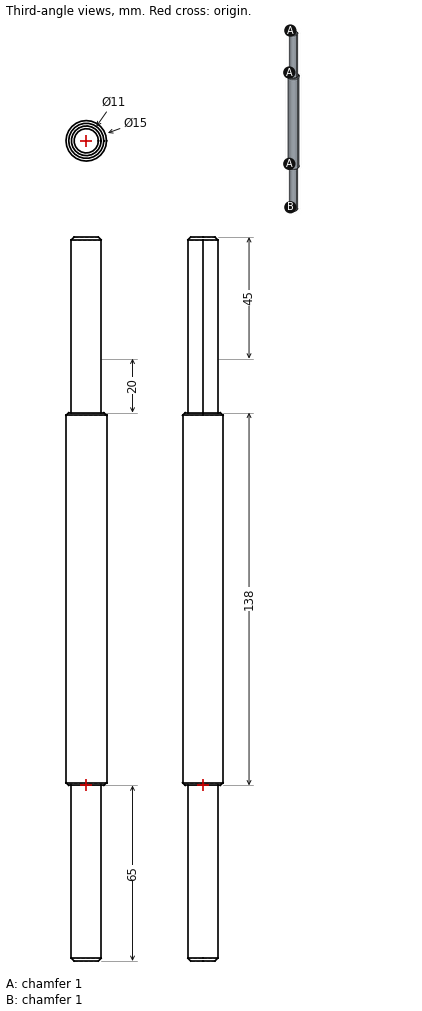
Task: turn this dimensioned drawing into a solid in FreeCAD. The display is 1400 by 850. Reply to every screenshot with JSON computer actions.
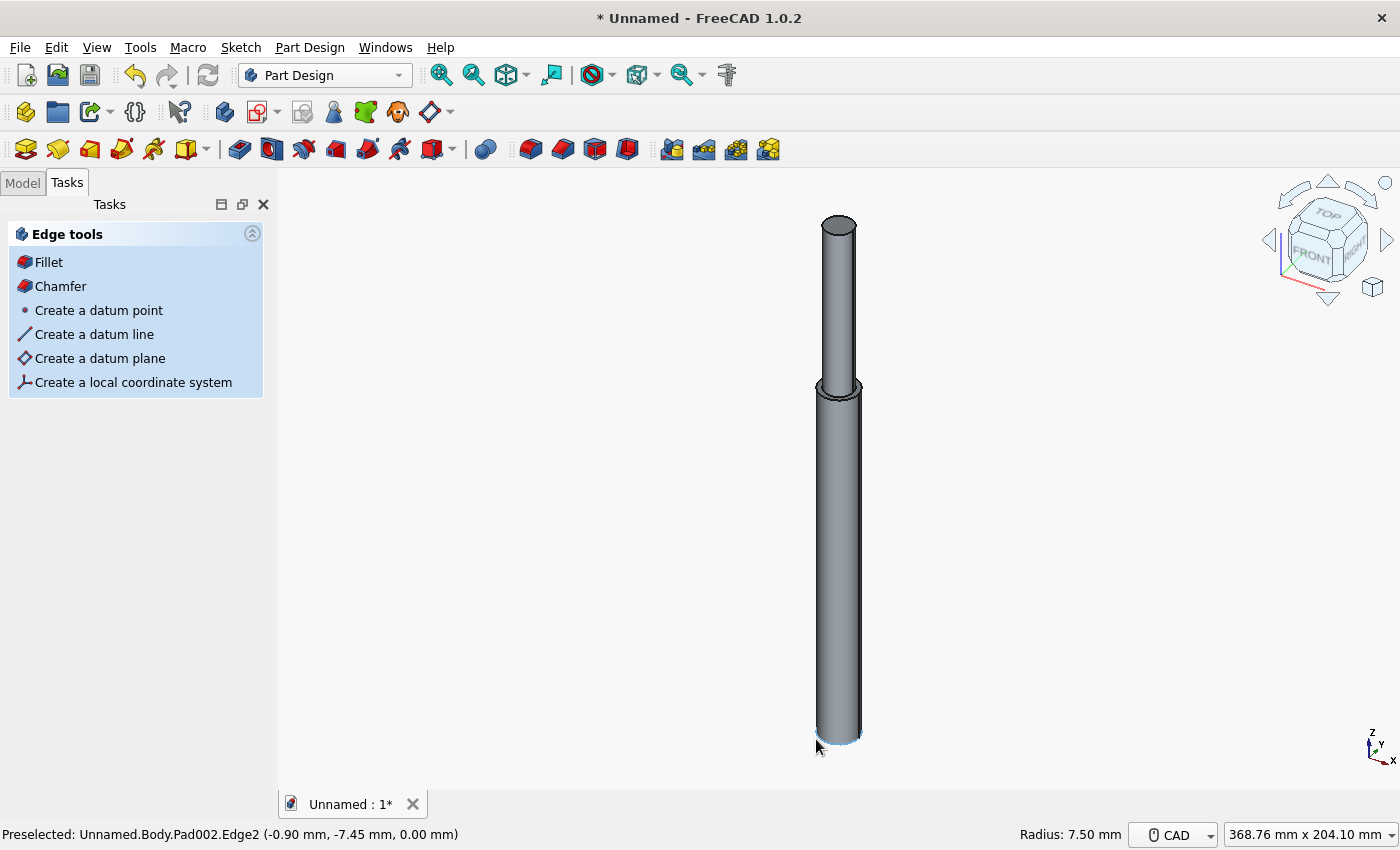
{"action": "left_click", "coordinate": [816, 388], "text": "ctrl"}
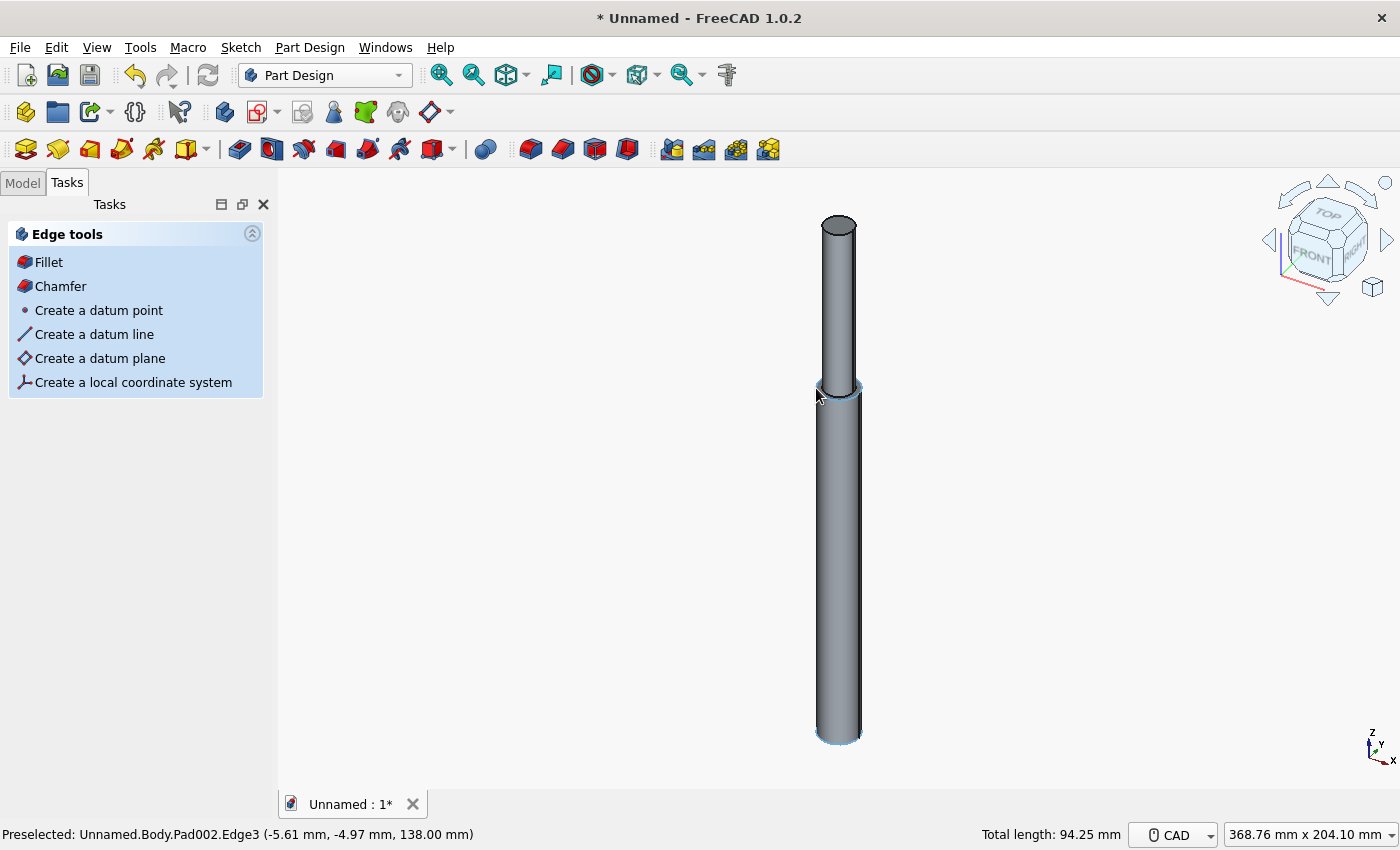
{"action": "left_click", "coordinate": [825, 220], "text": "ctrl"}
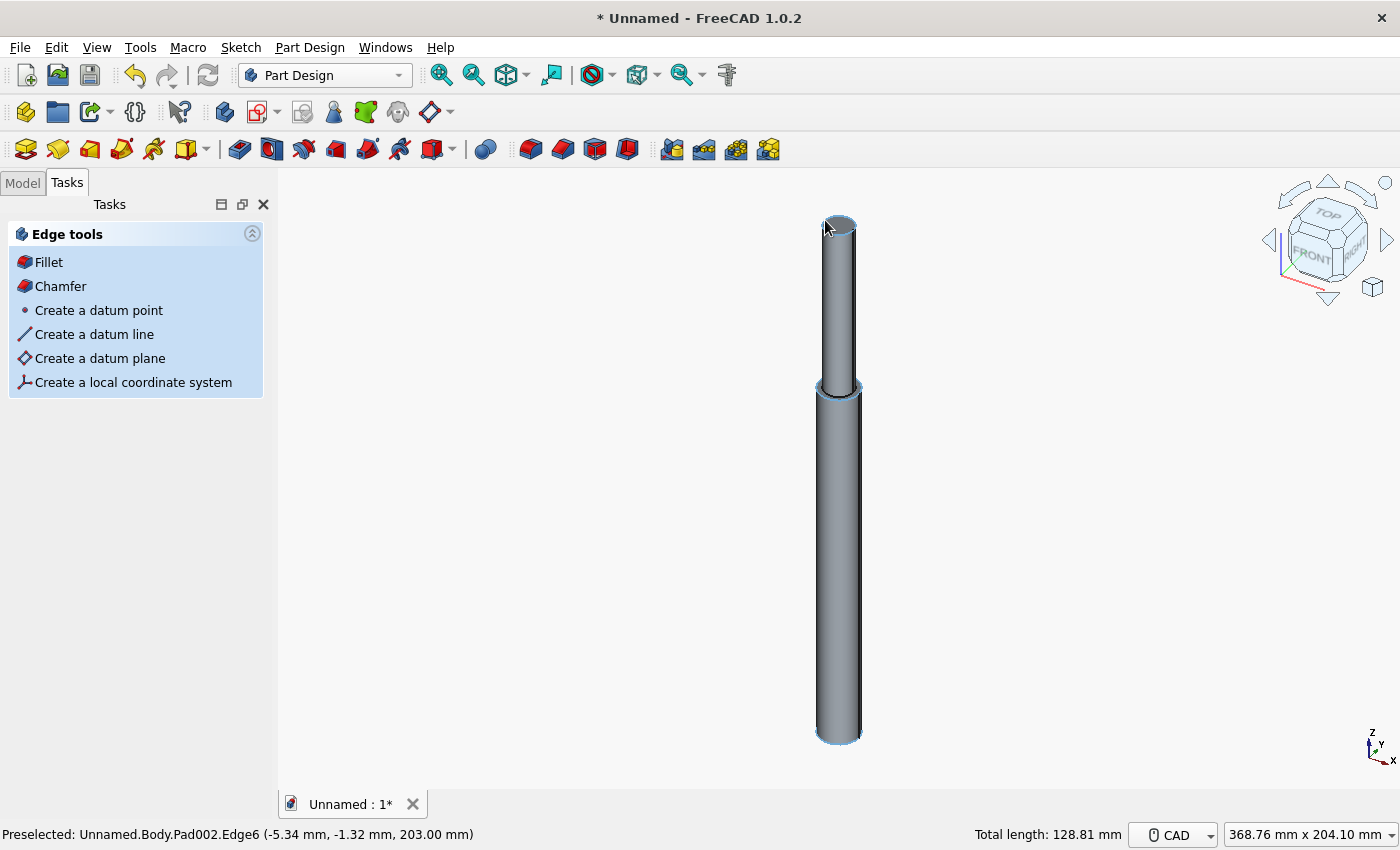
{"action": "left_click", "coordinate": [564, 150]}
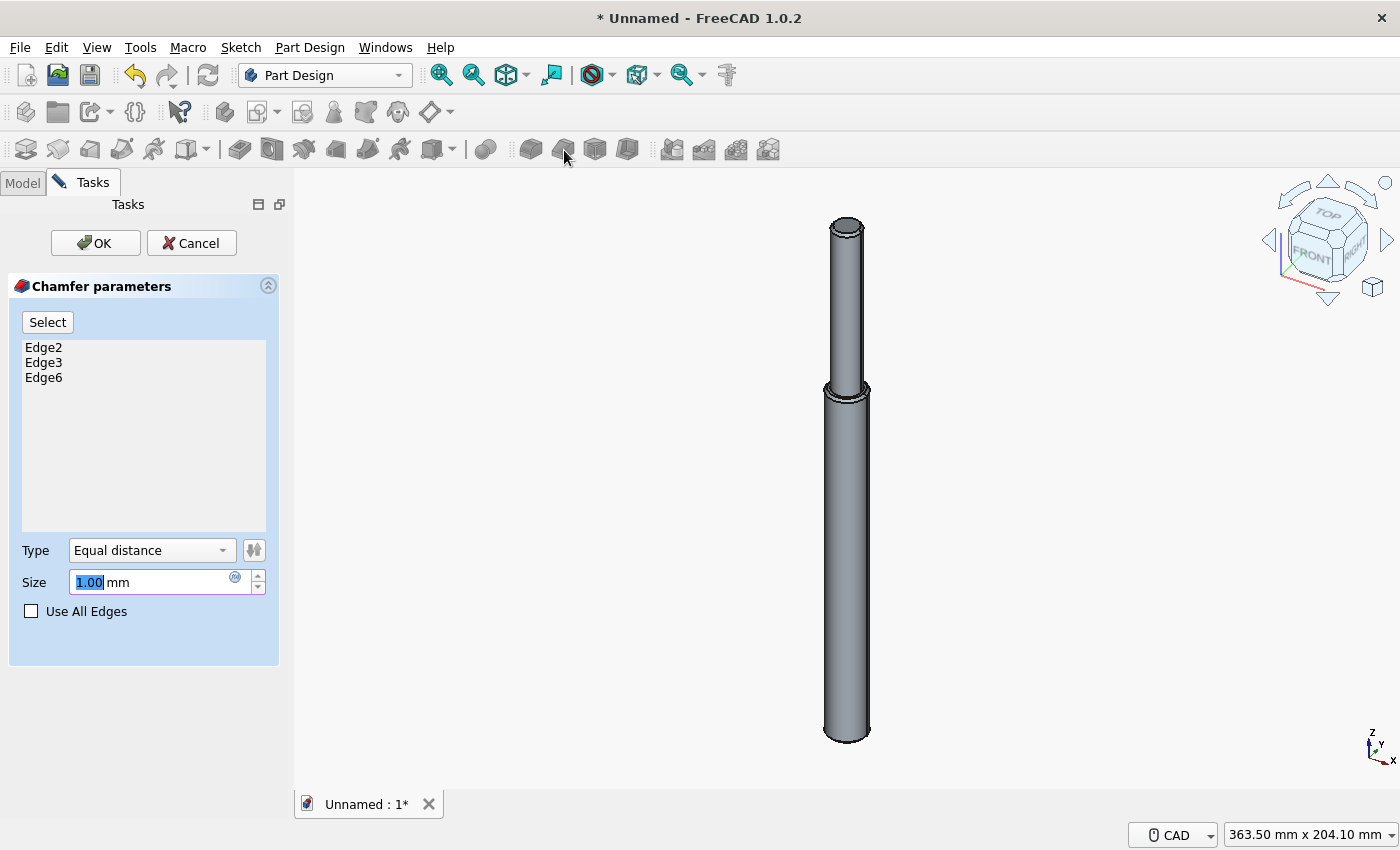
{"action": "type", "text": "1"}
{"action": "key", "text": "Tab"}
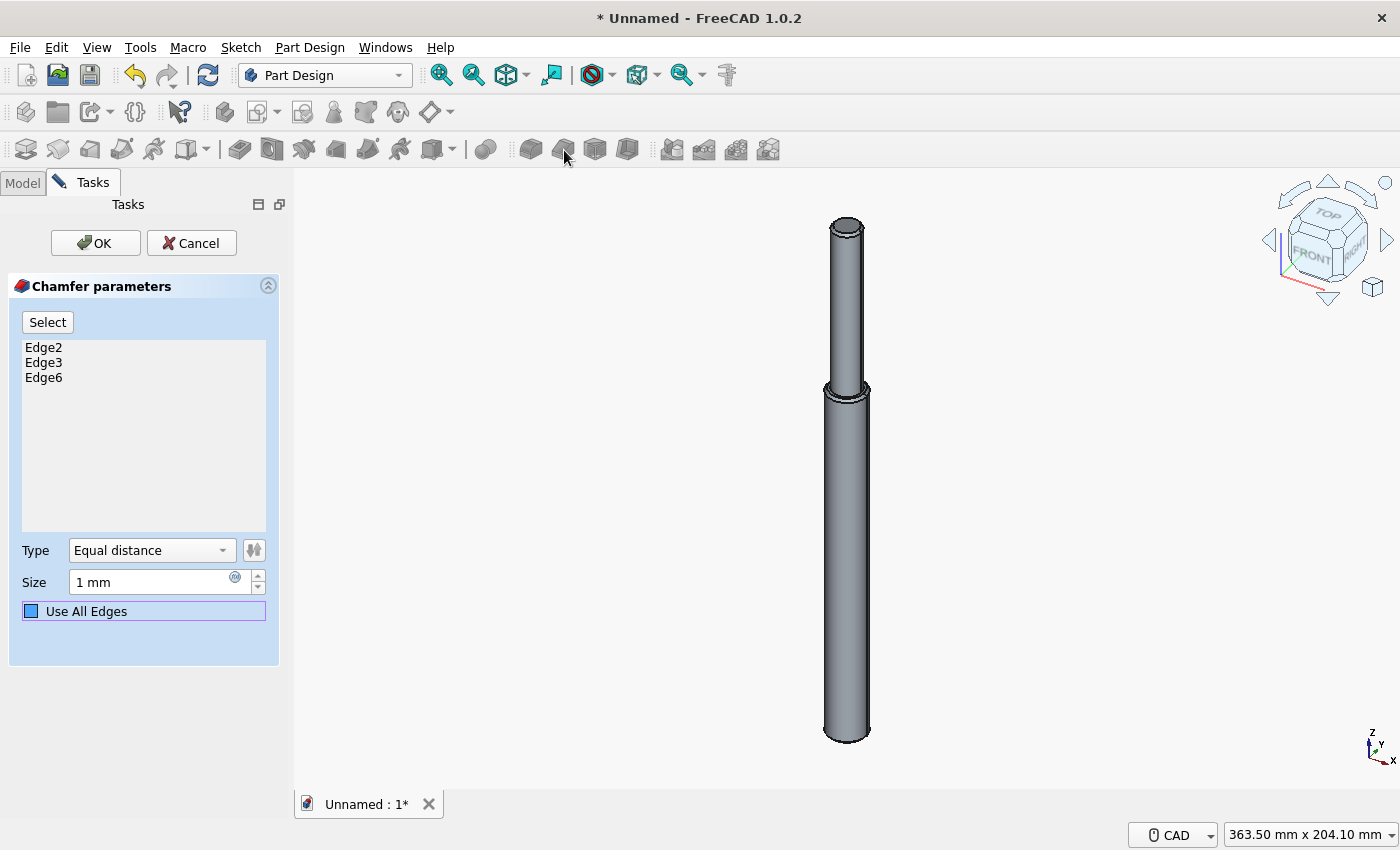
{"action": "left_click", "coordinate": [96, 243]}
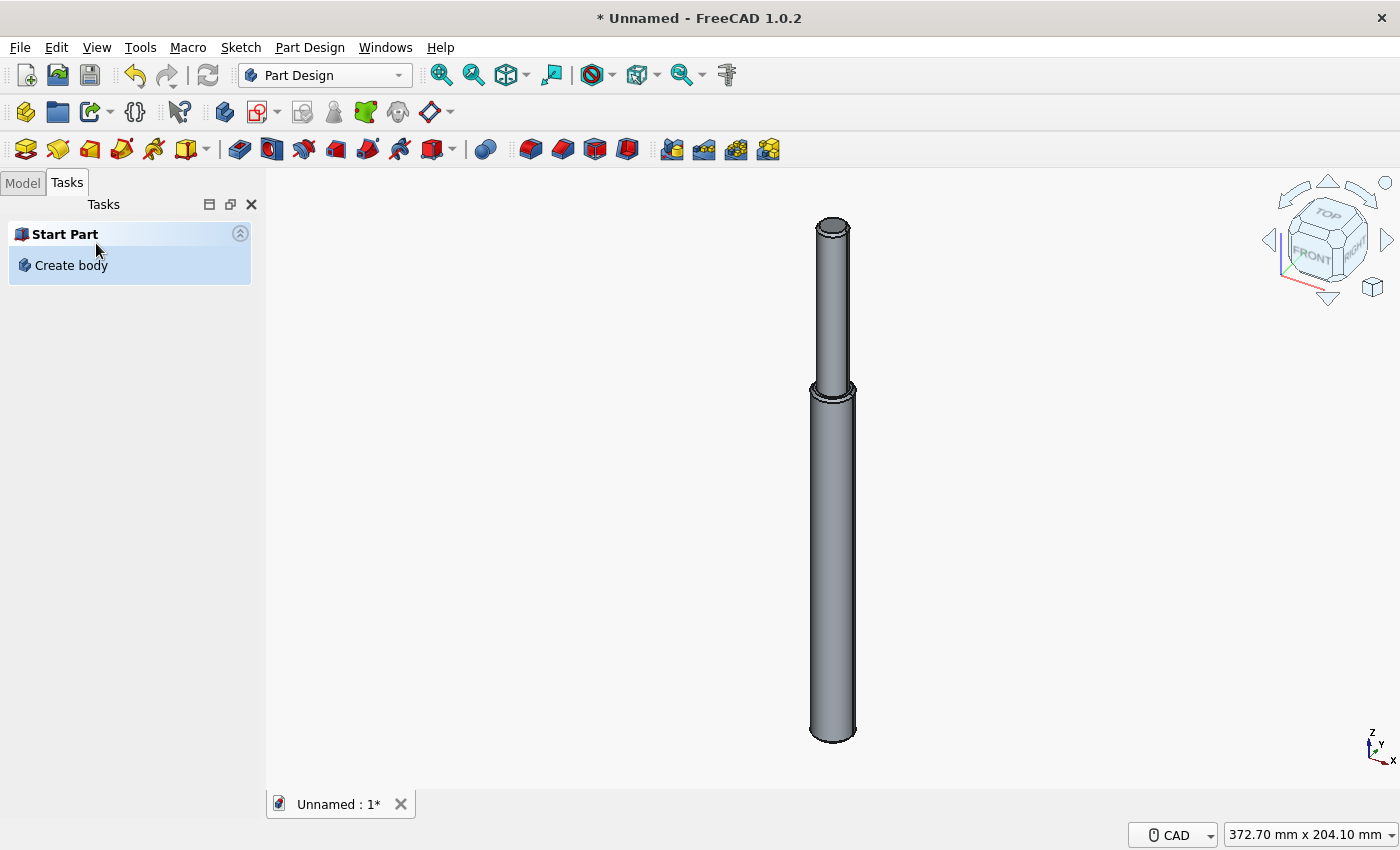
{"action": "left_click", "coordinate": [23, 182]}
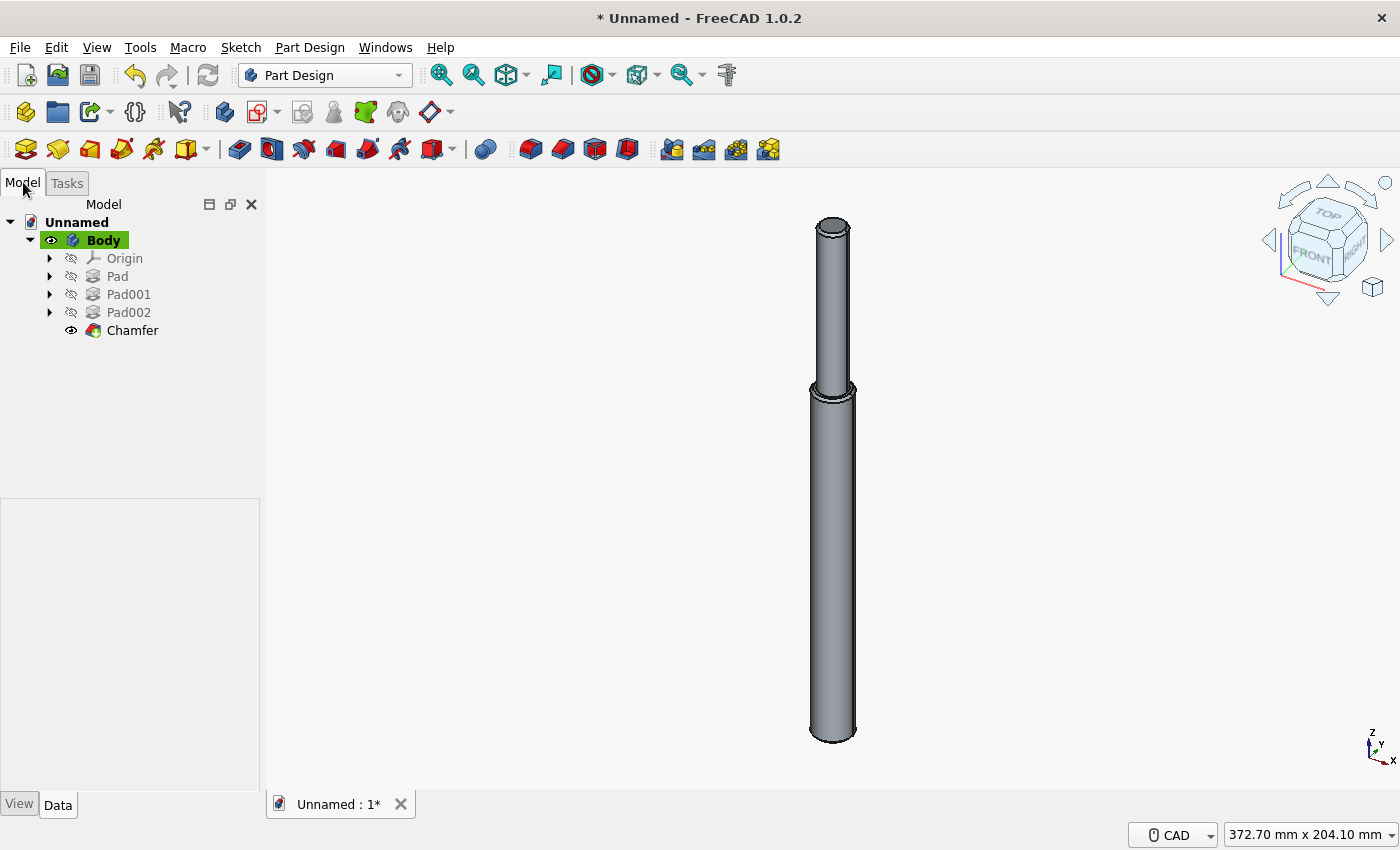
{"action": "left_click", "coordinate": [50, 258]}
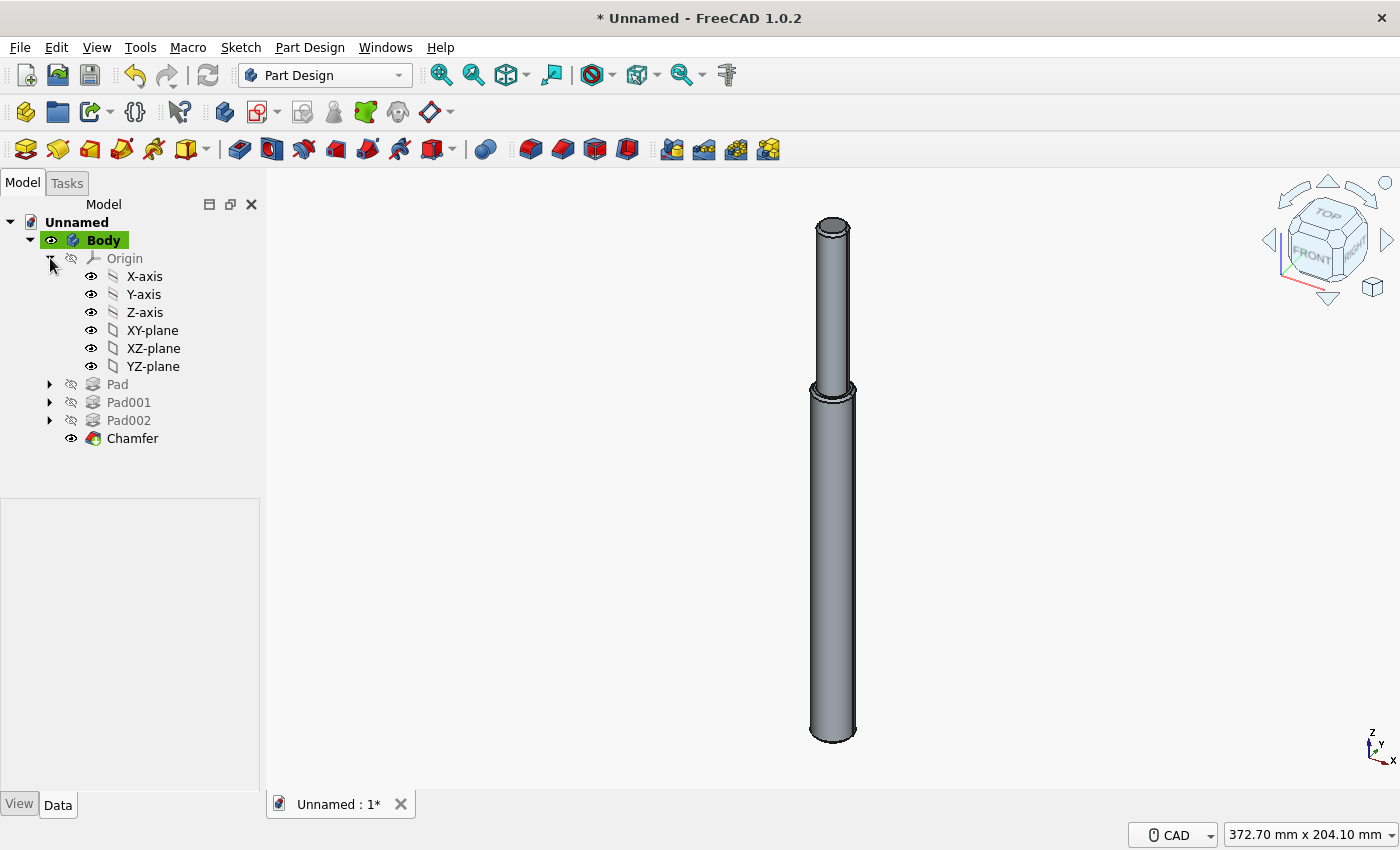
{"action": "left_click", "coordinate": [136, 330]}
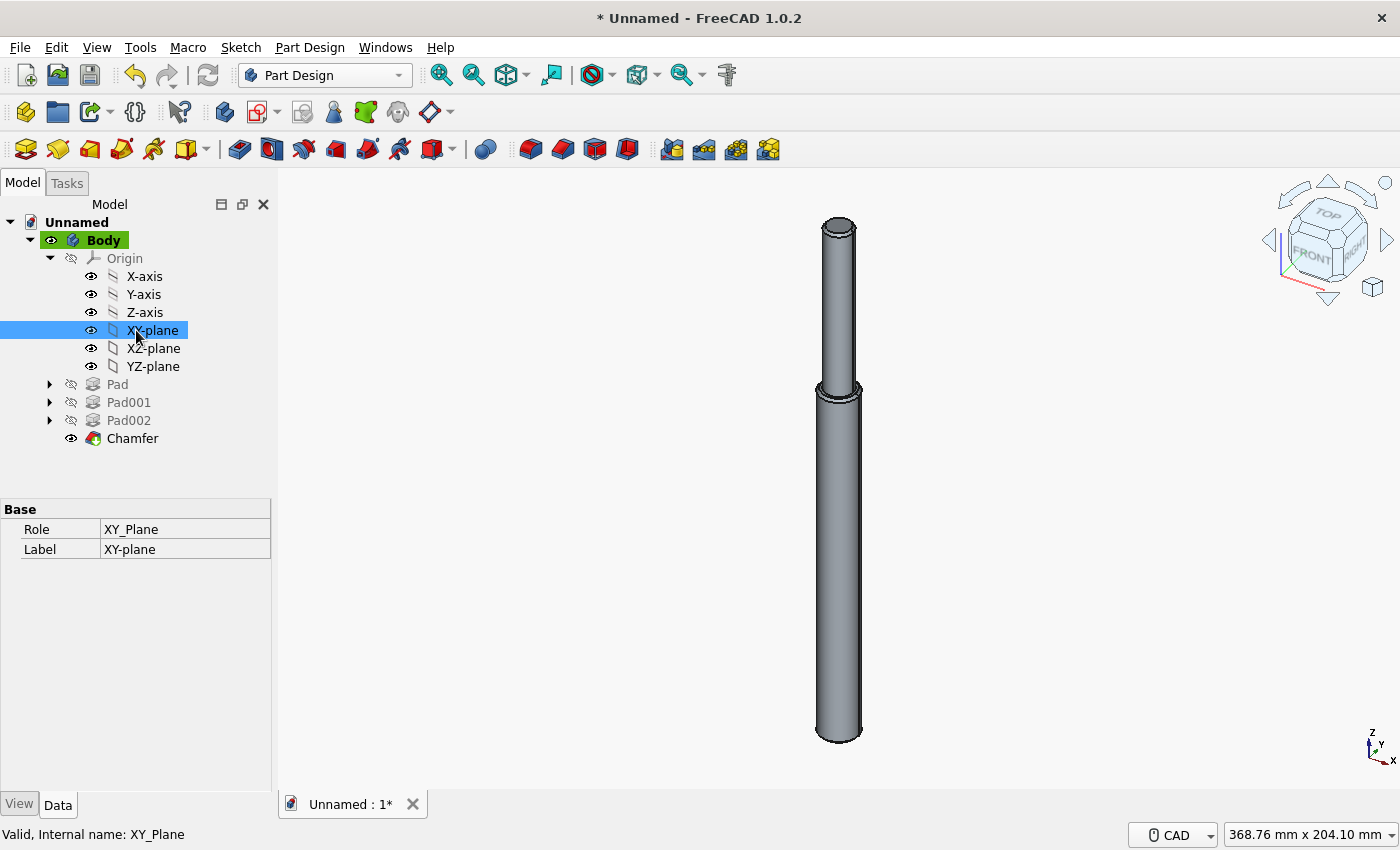
{"action": "left_click", "coordinate": [430, 112]}